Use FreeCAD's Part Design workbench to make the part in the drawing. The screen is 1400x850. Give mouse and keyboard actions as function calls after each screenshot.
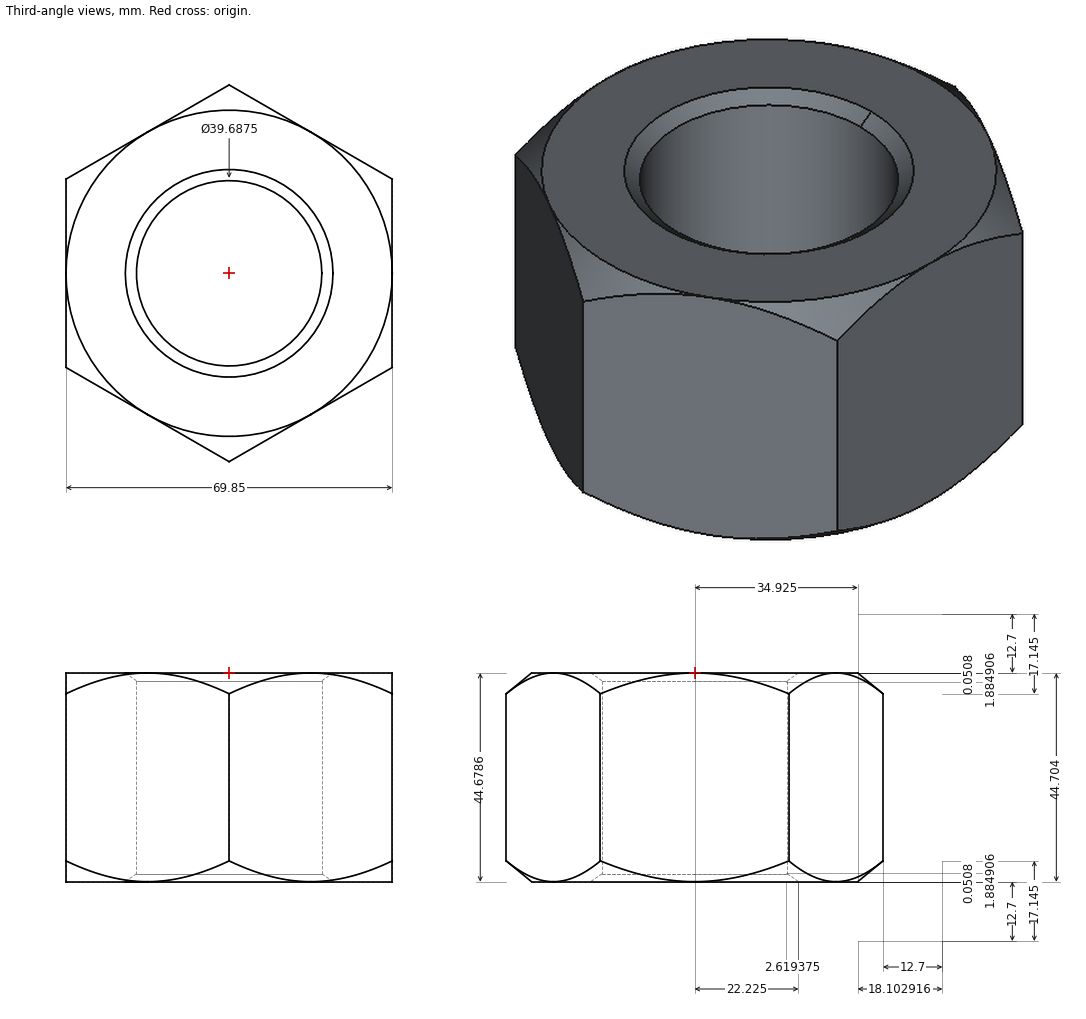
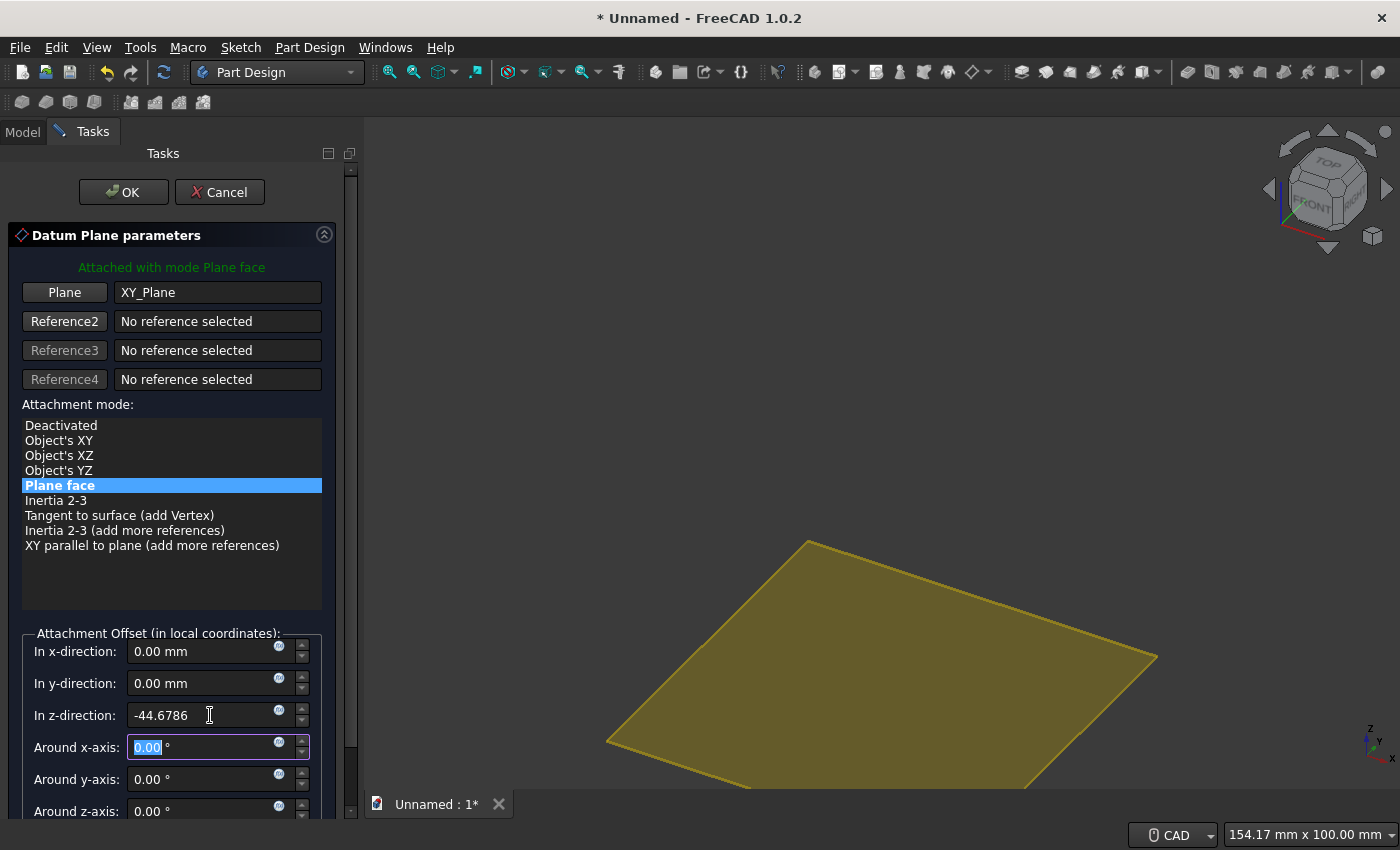
click(124, 192)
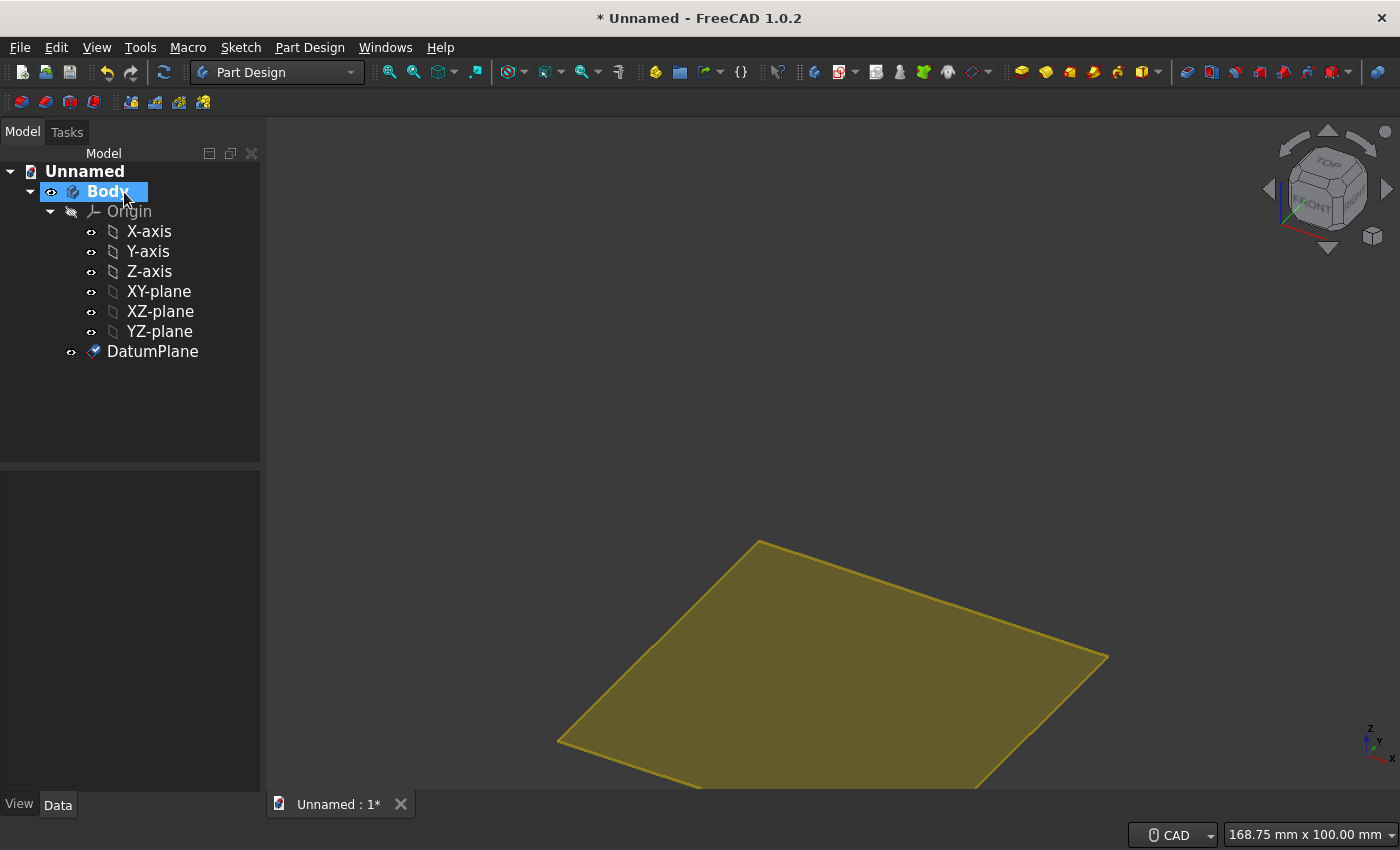
click(116, 352)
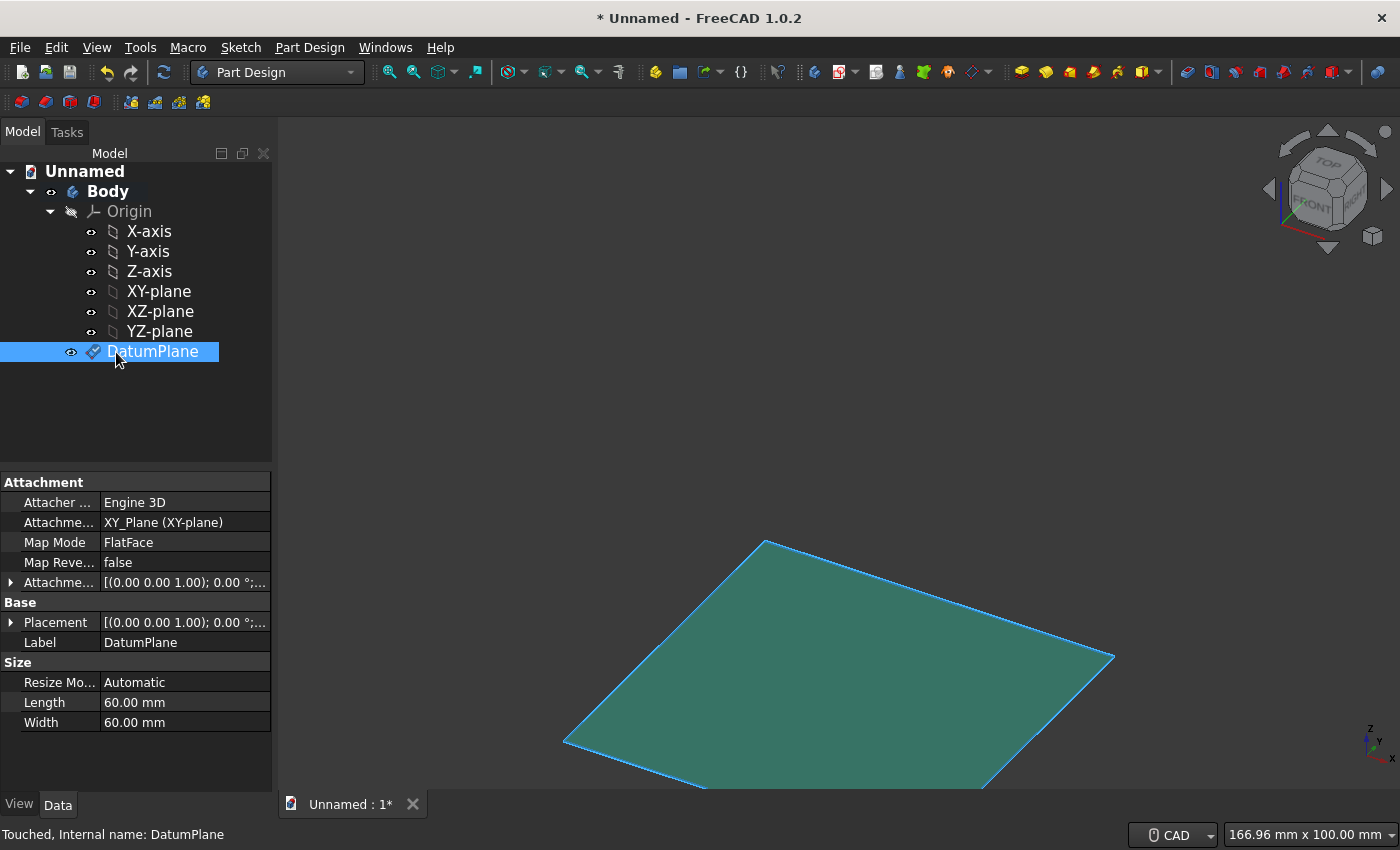
click(840, 72)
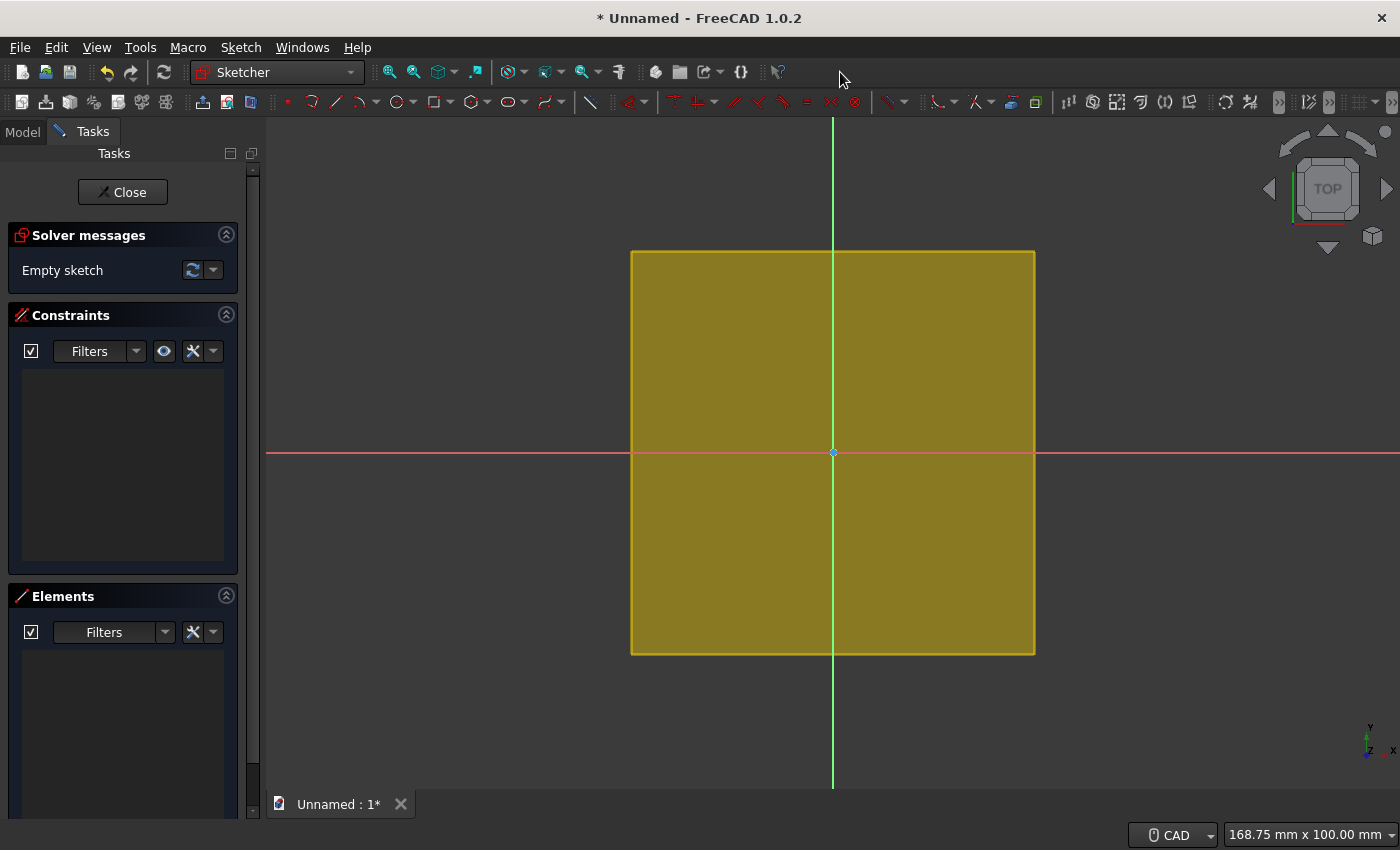
click(472, 102)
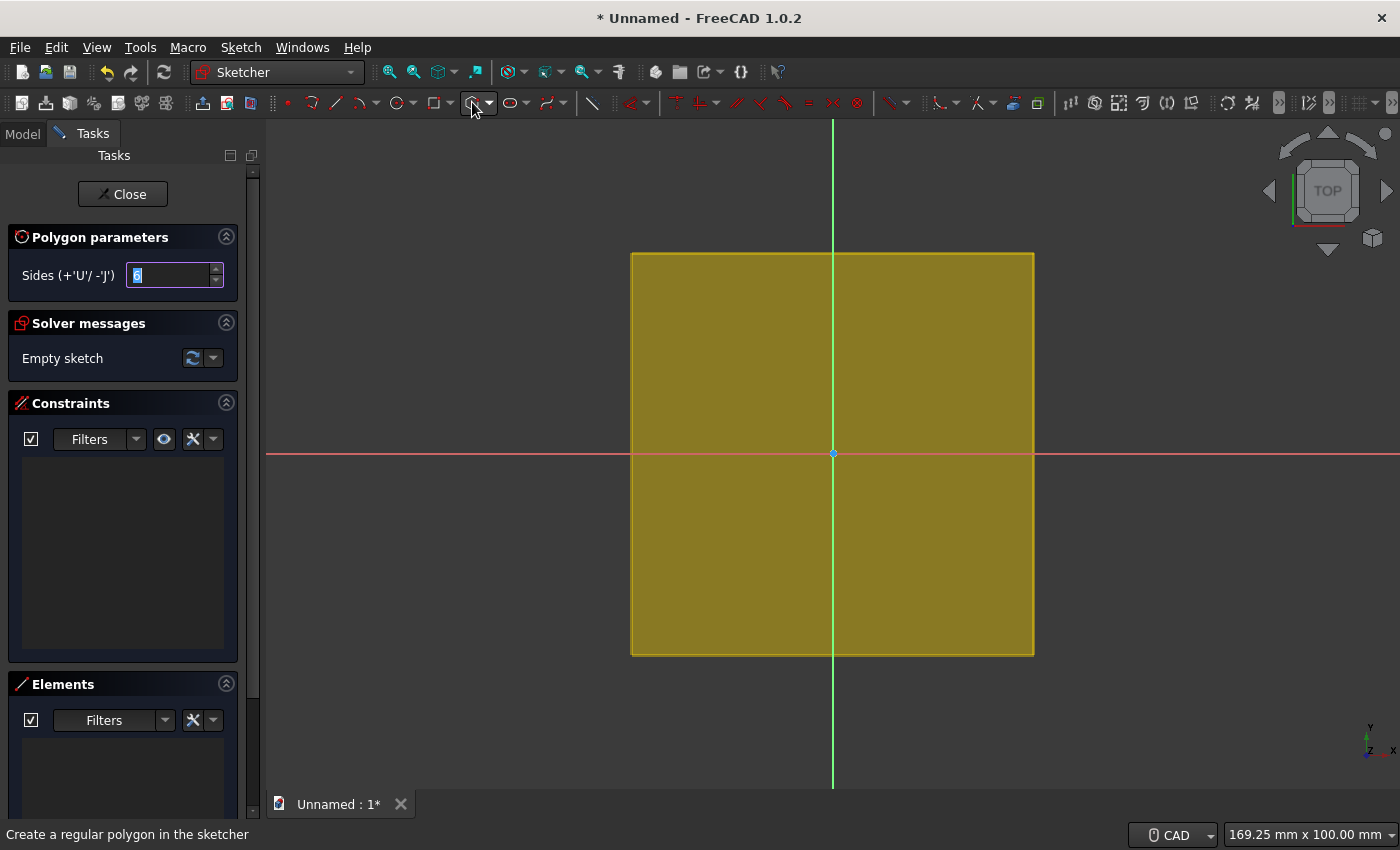
click(833, 454)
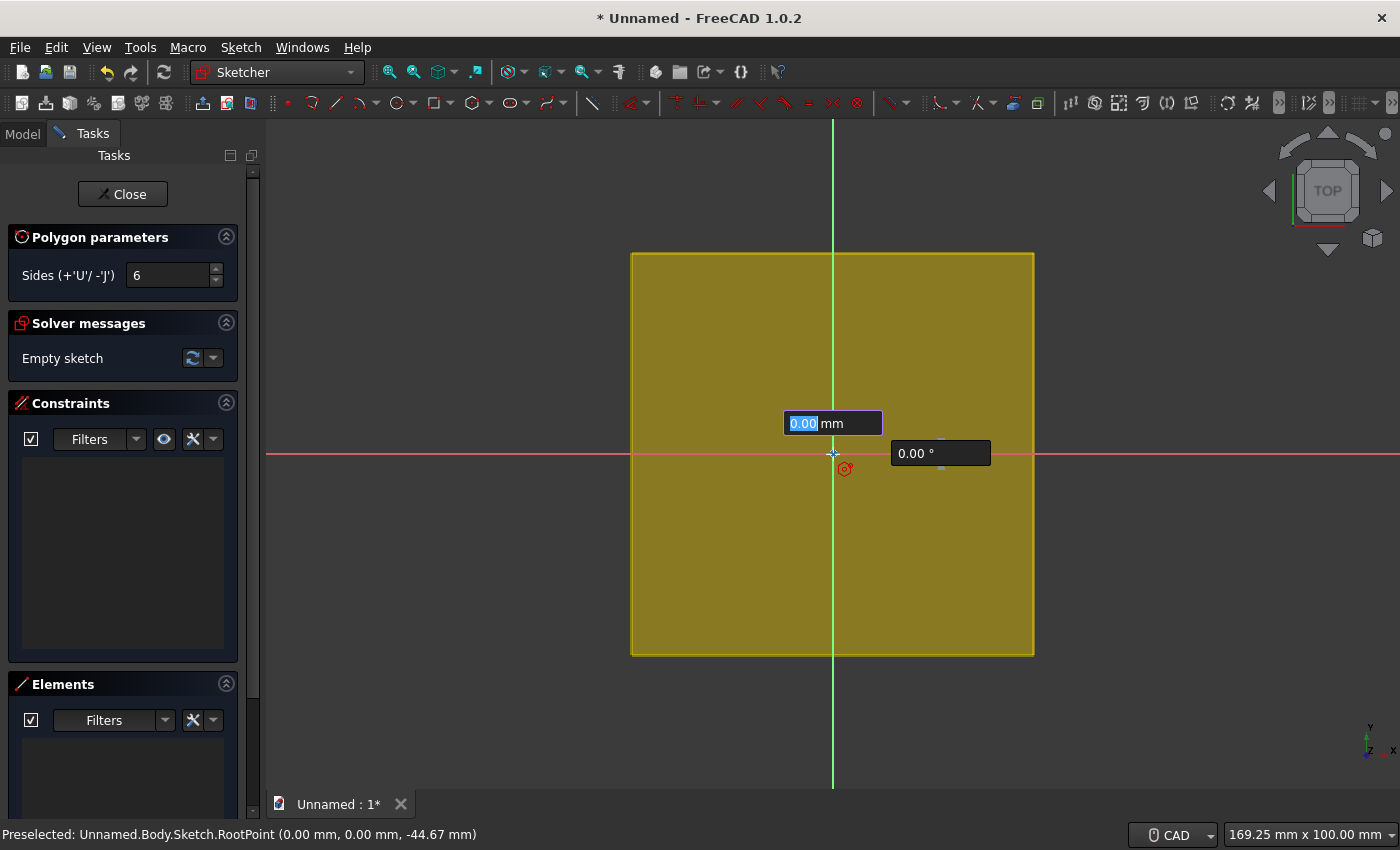
click(833, 184)
key(Escape)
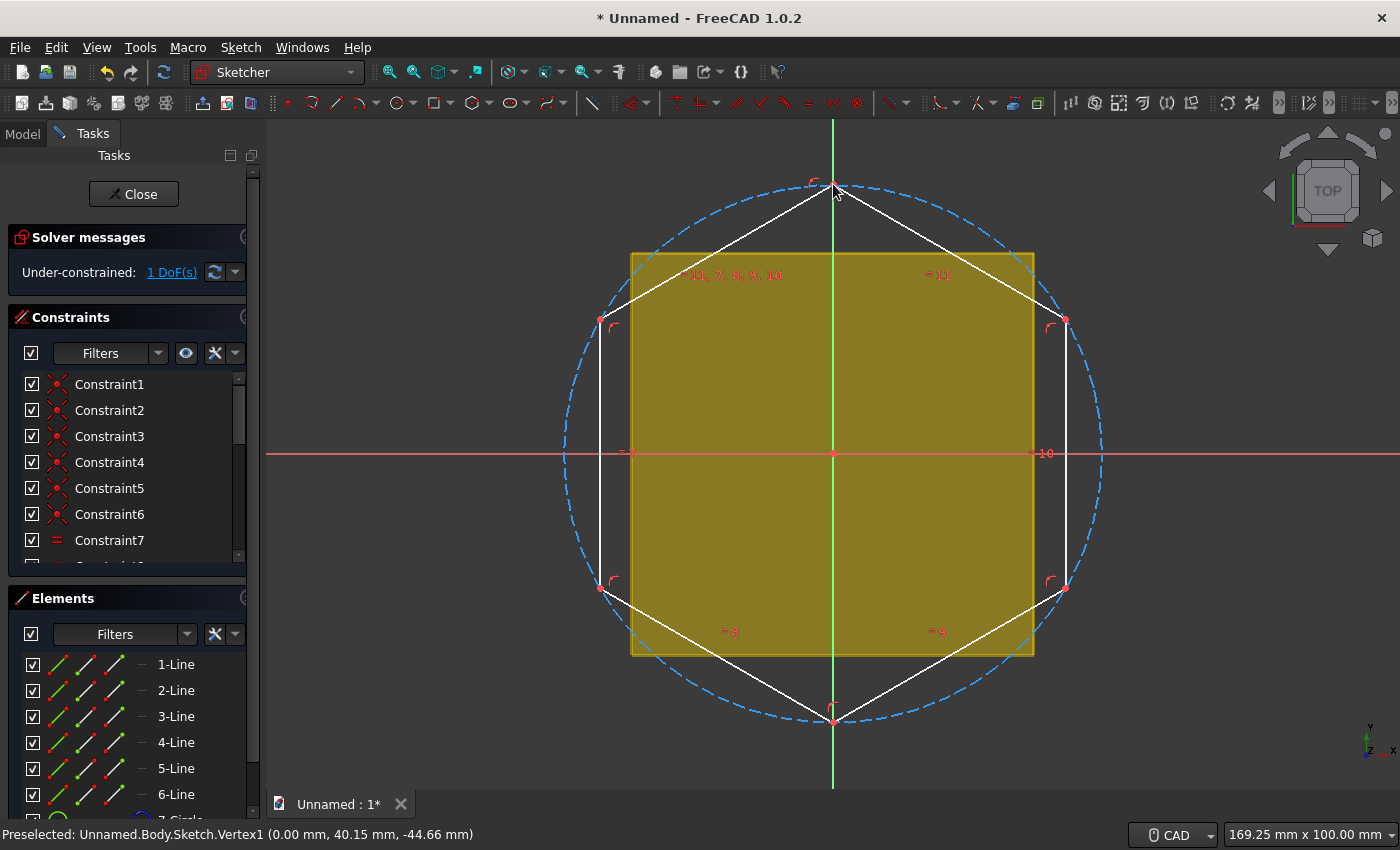
click(398, 104)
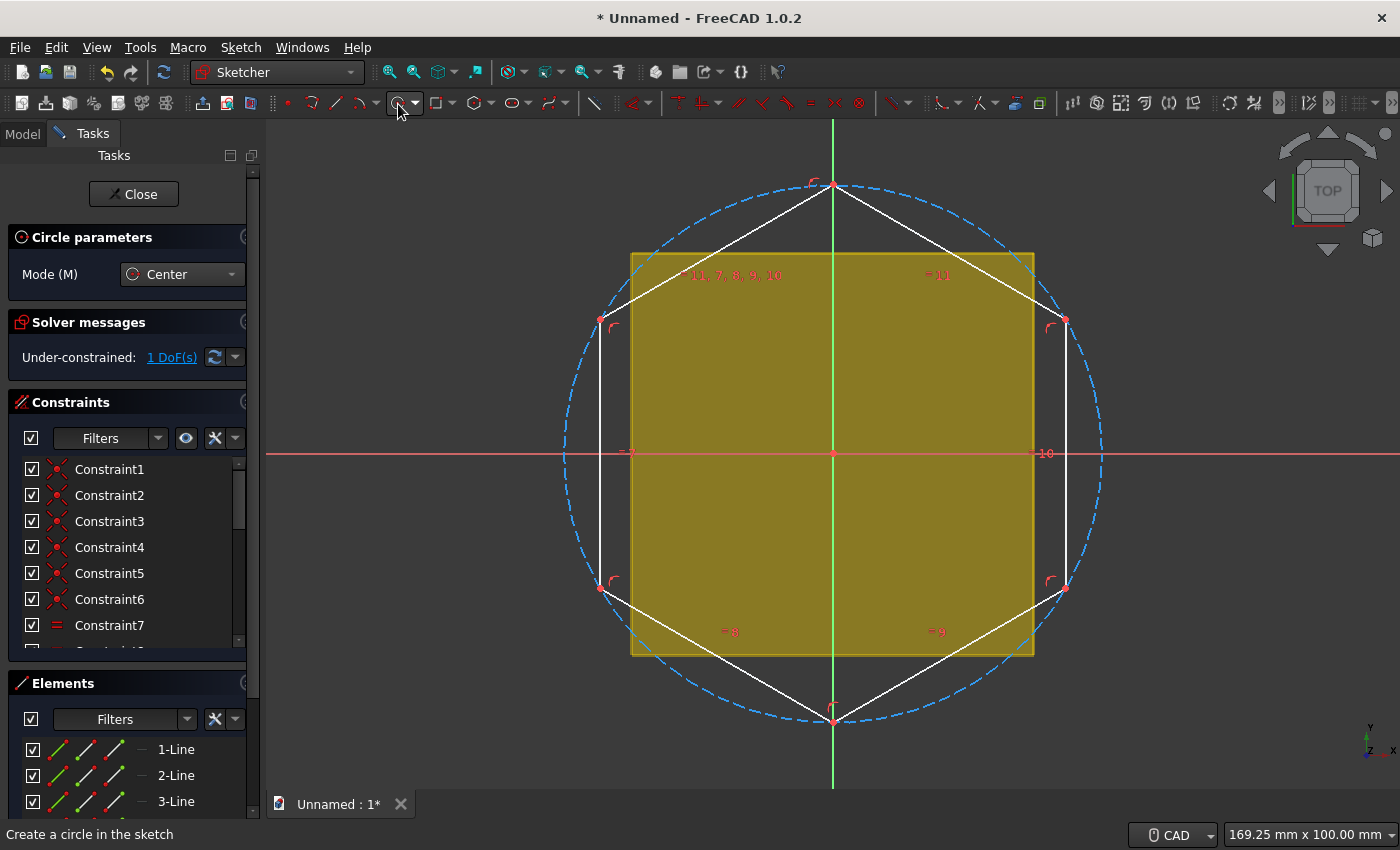
click(833, 454)
move(927, 360)